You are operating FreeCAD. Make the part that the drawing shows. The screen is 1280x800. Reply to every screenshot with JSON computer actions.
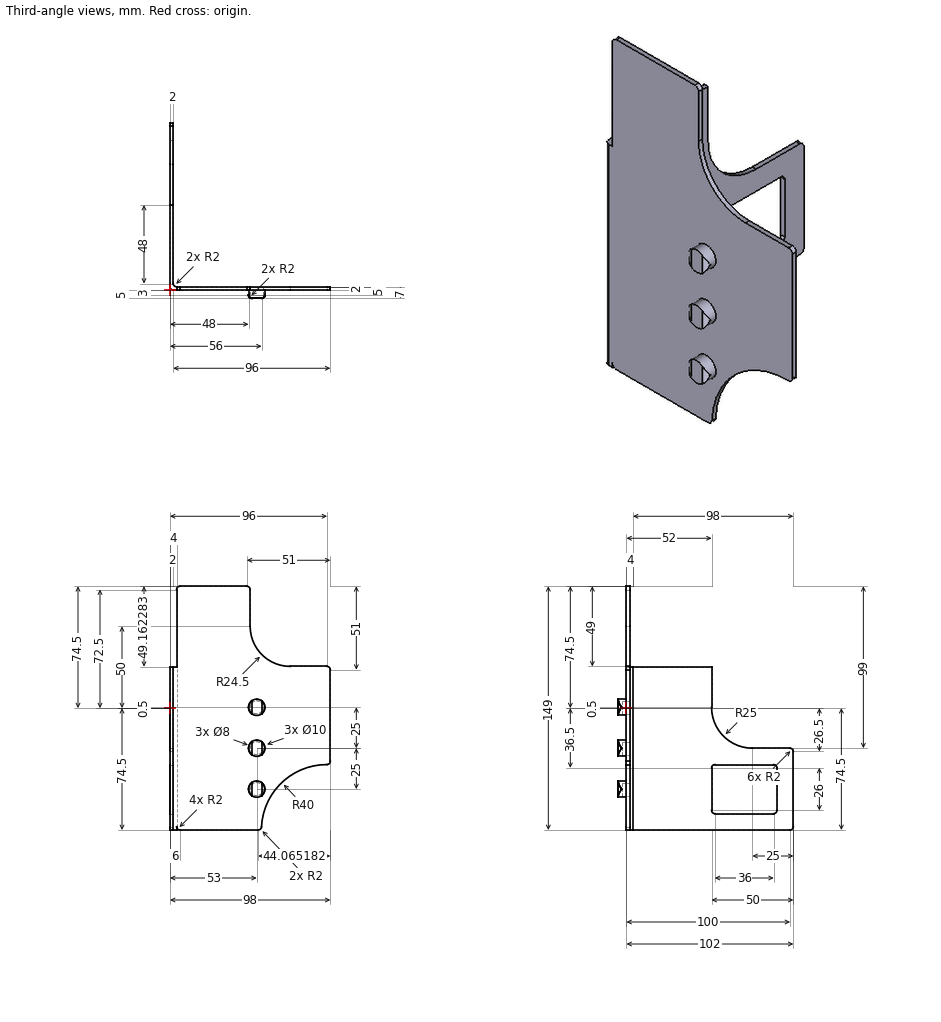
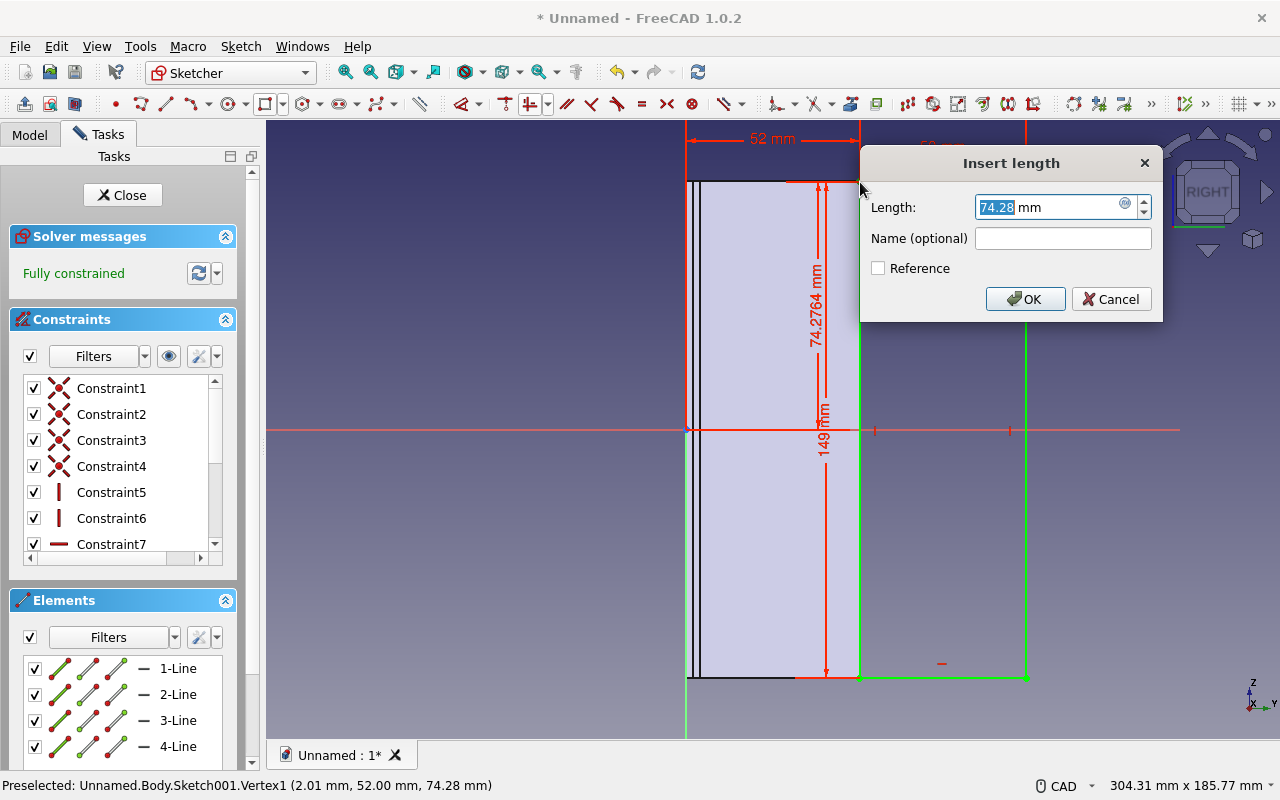
{"action": "type", "text": "74.5"}
{"action": "key", "text": "Return"}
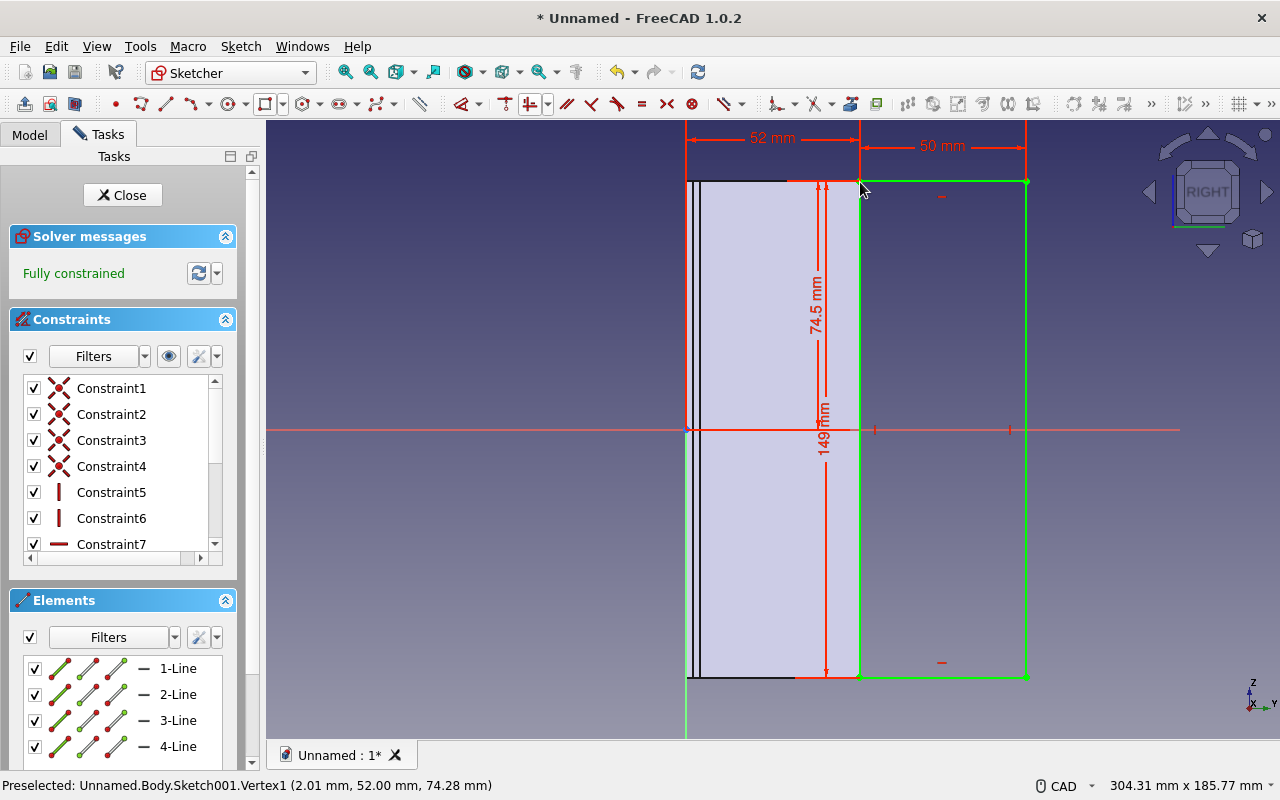
{"action": "left_click", "coordinate": [123, 195]}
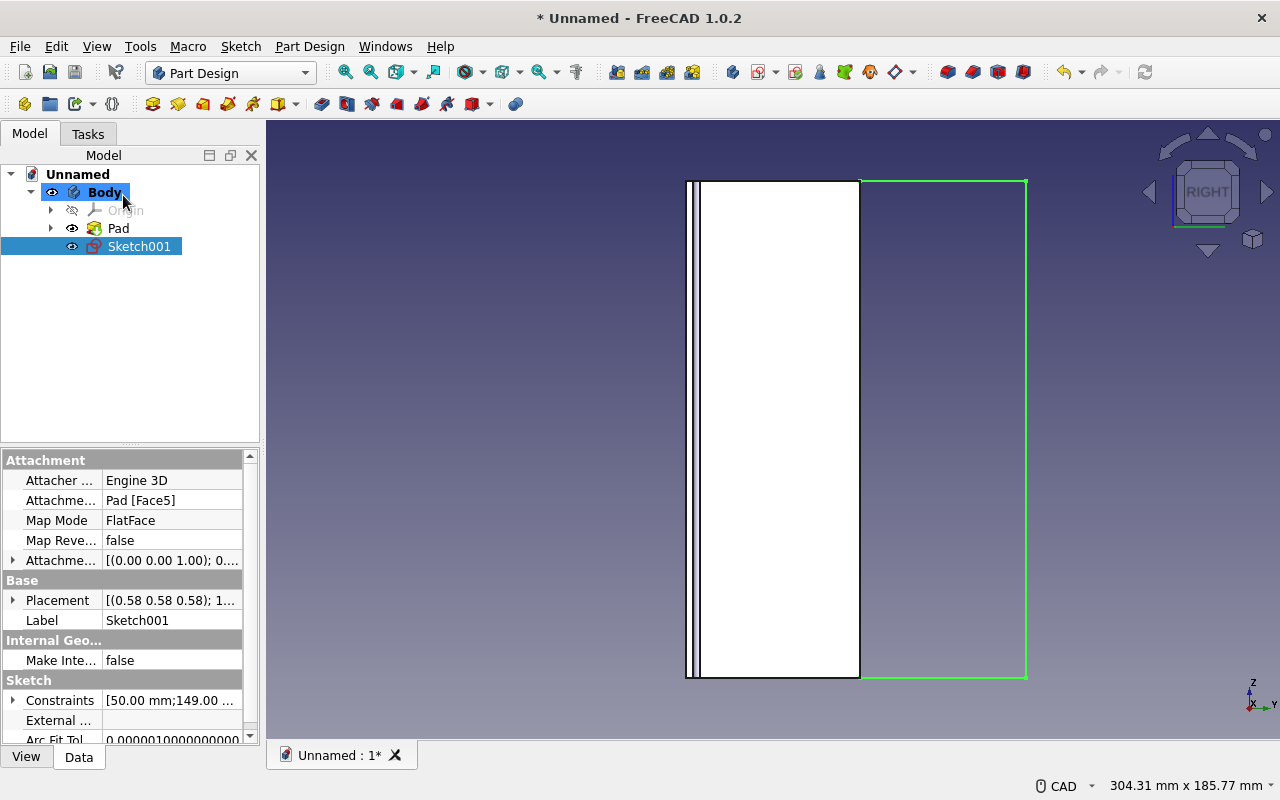
{"action": "left_click", "coordinate": [153, 104]}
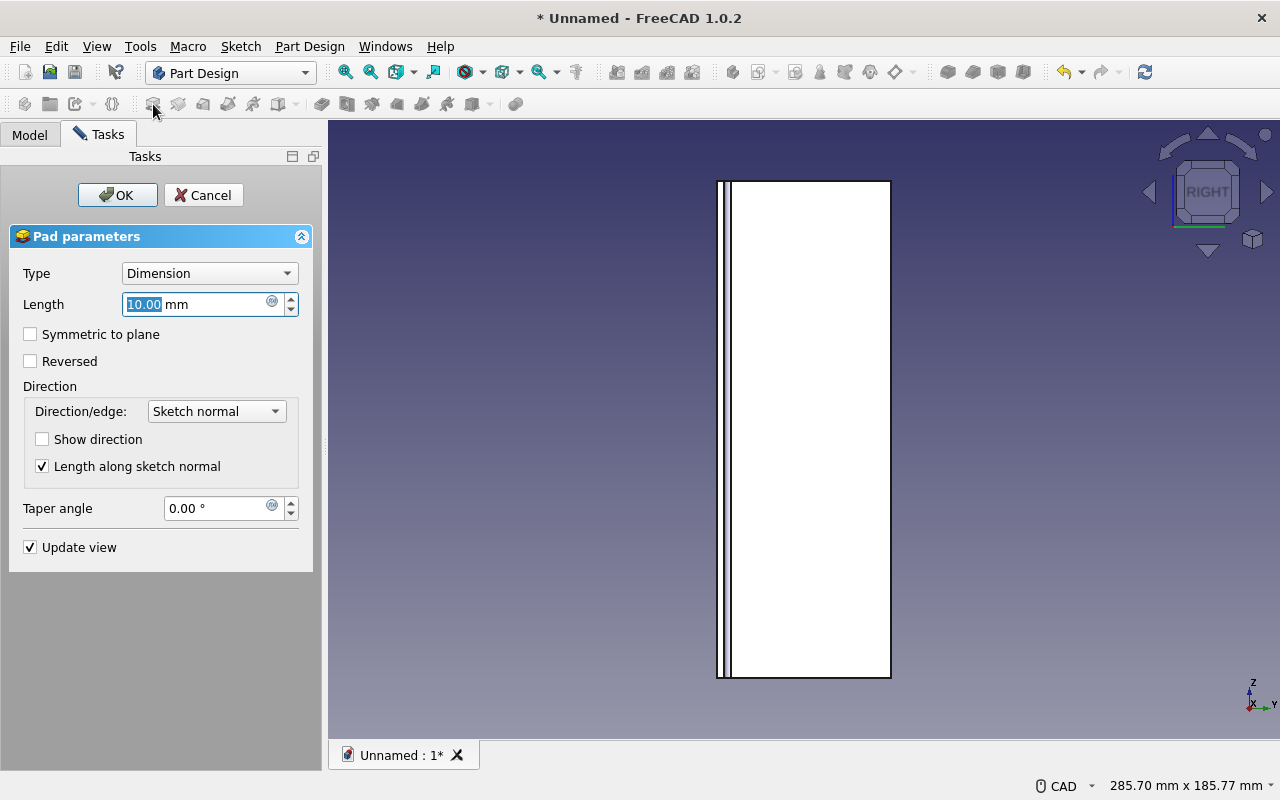
{"action": "type", "text": "2"}
{"action": "key", "text": "Tab"}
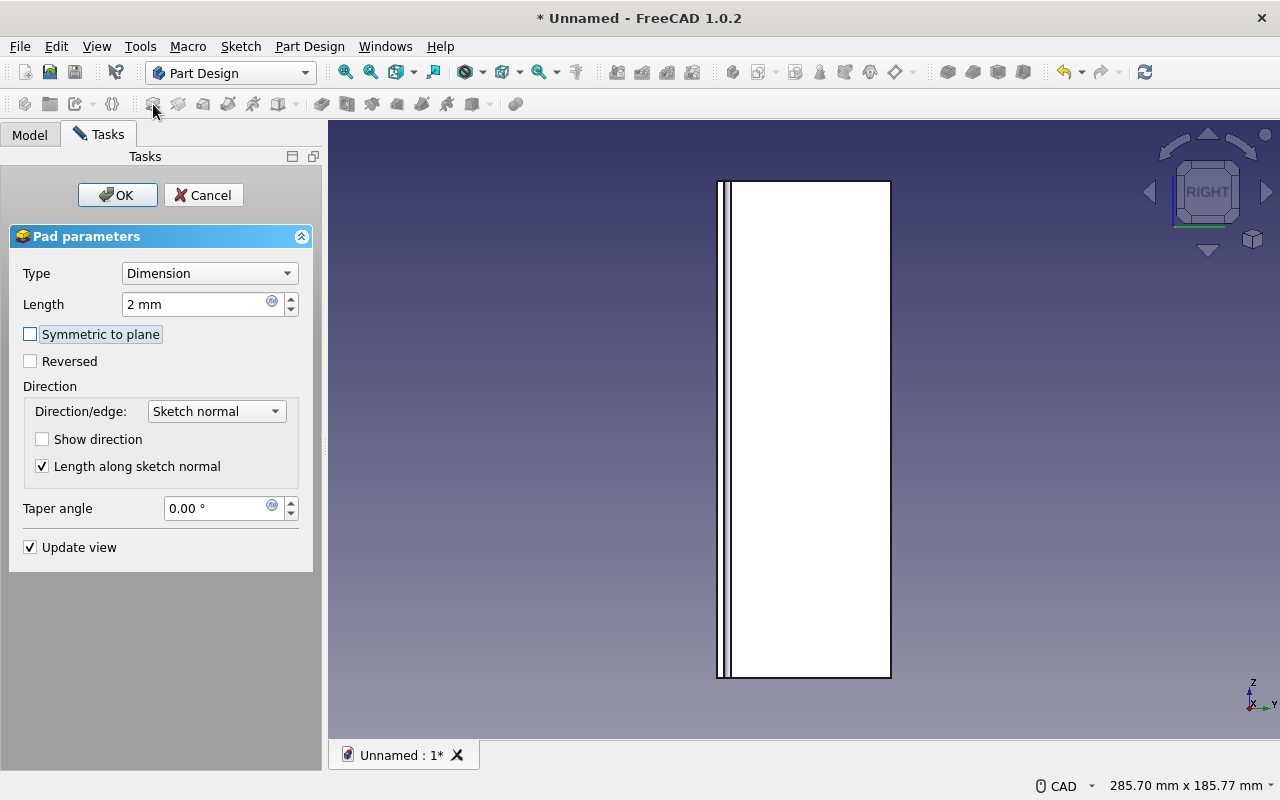
{"action": "left_click", "coordinate": [31, 361]}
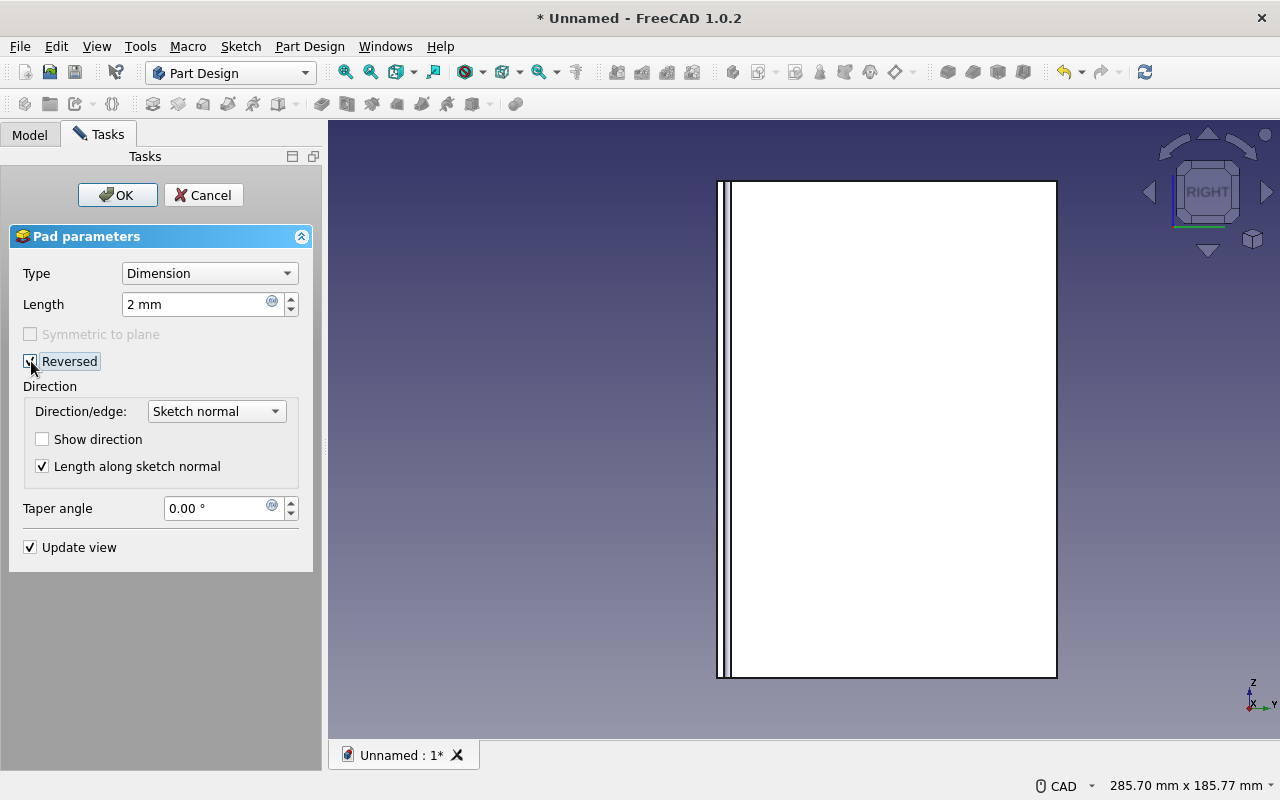
{"action": "left_click", "coordinate": [118, 195]}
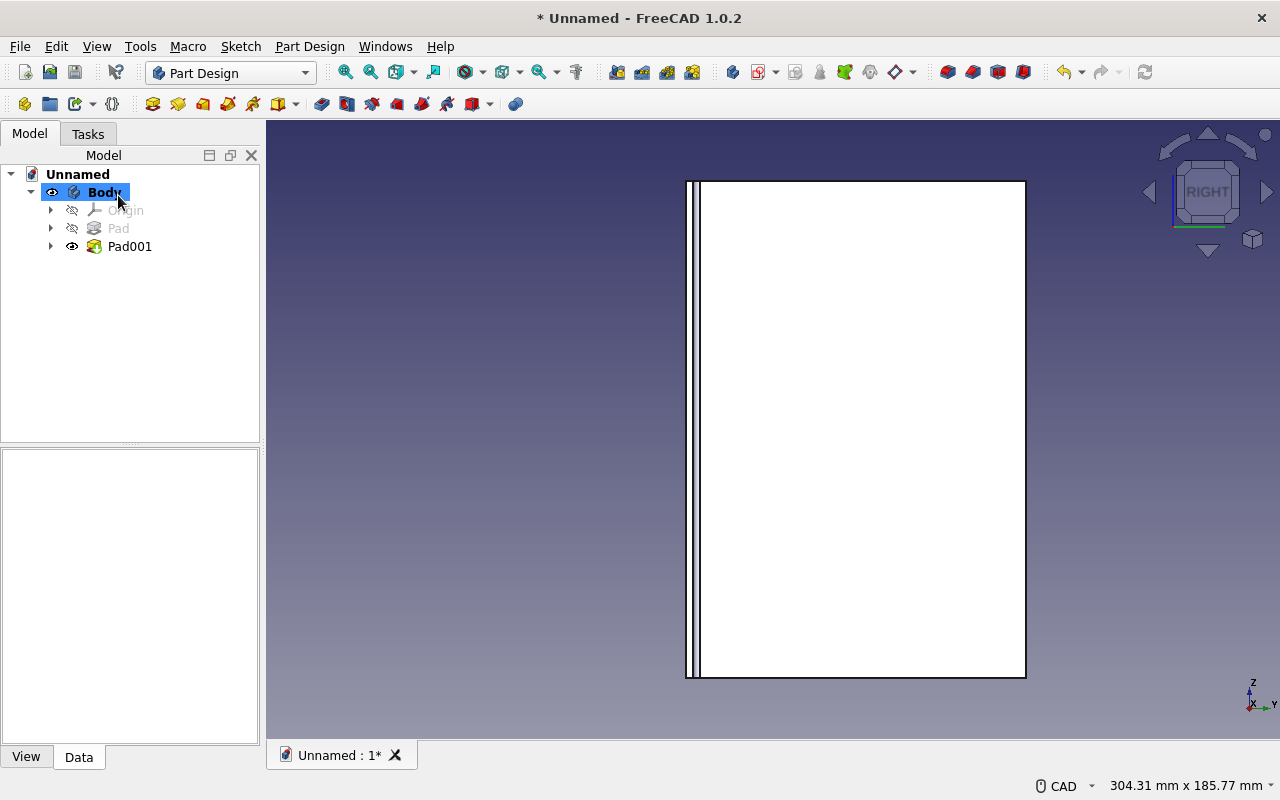
{"action": "left_click", "coordinate": [863, 358]}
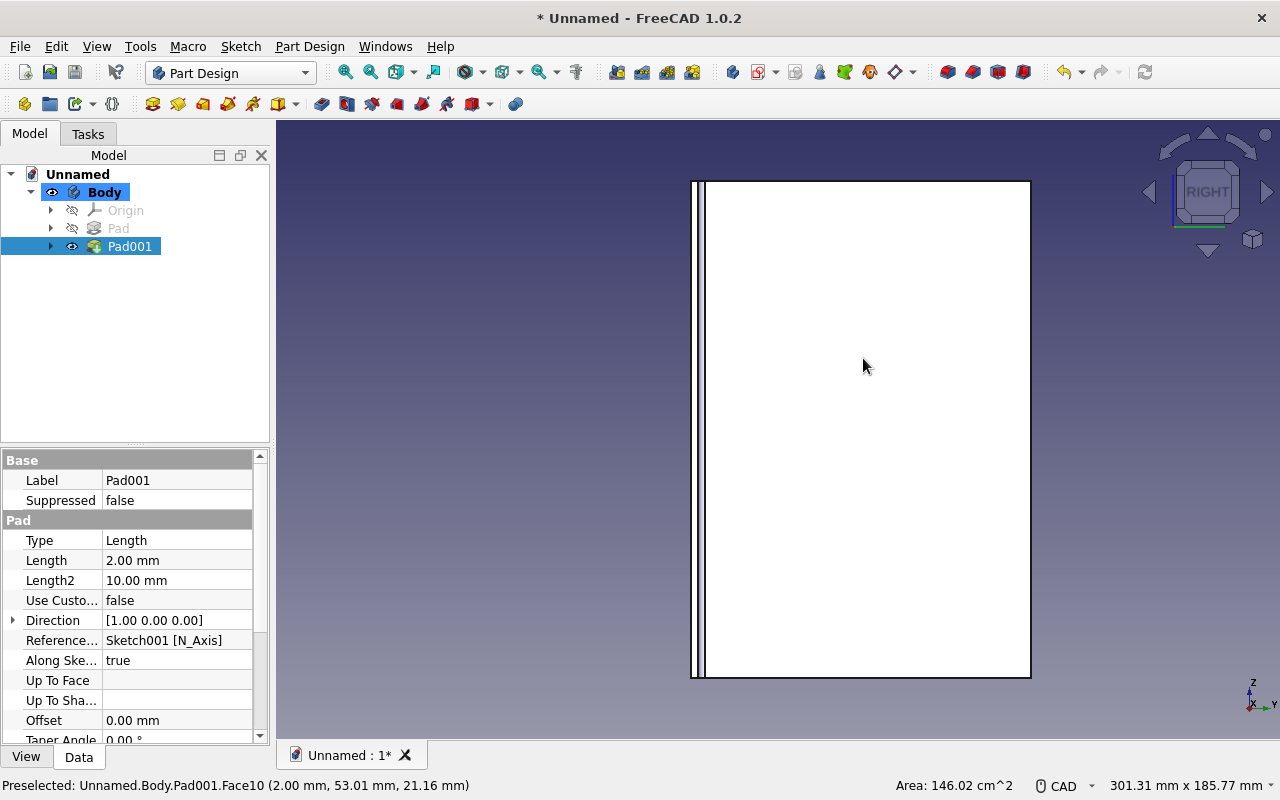
{"action": "left_click", "coordinate": [758, 72]}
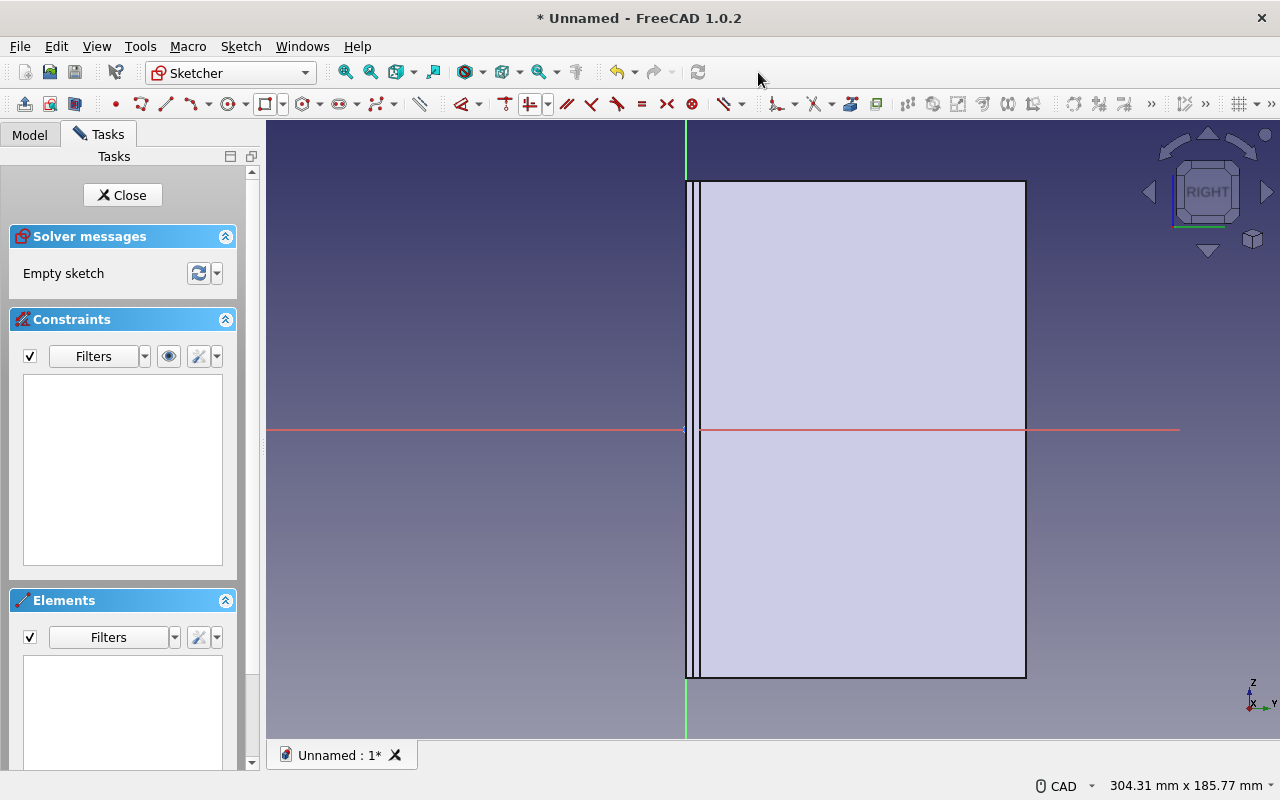
{"action": "left_click", "coordinate": [141, 104]}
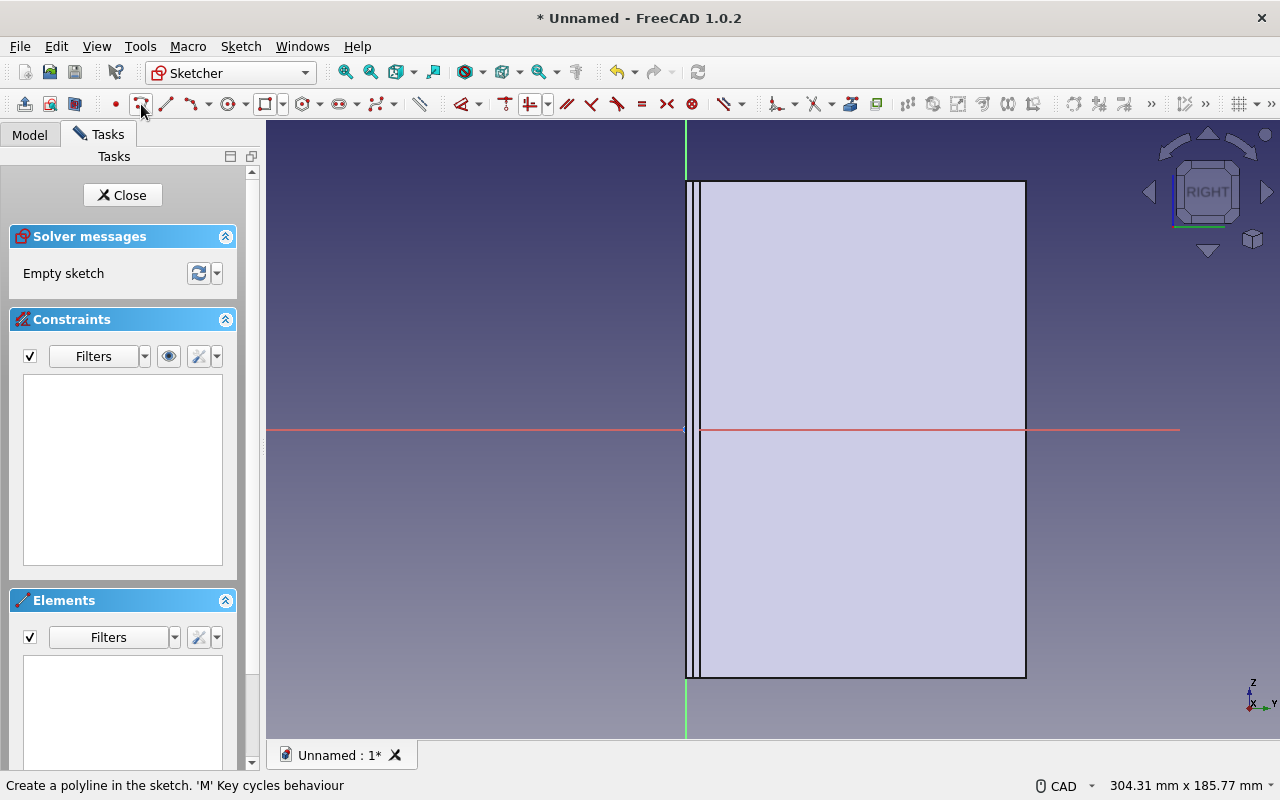
{"action": "left_click", "coordinate": [943, 511]}
{"action": "left_click", "coordinate": [1026, 511]}
{"action": "left_click", "coordinate": [1026, 181]}
{"action": "left_click", "coordinate": [700, 181]}
{"action": "left_click", "coordinate": [700, 345]}
{"action": "left_click", "coordinate": [860, 345]}